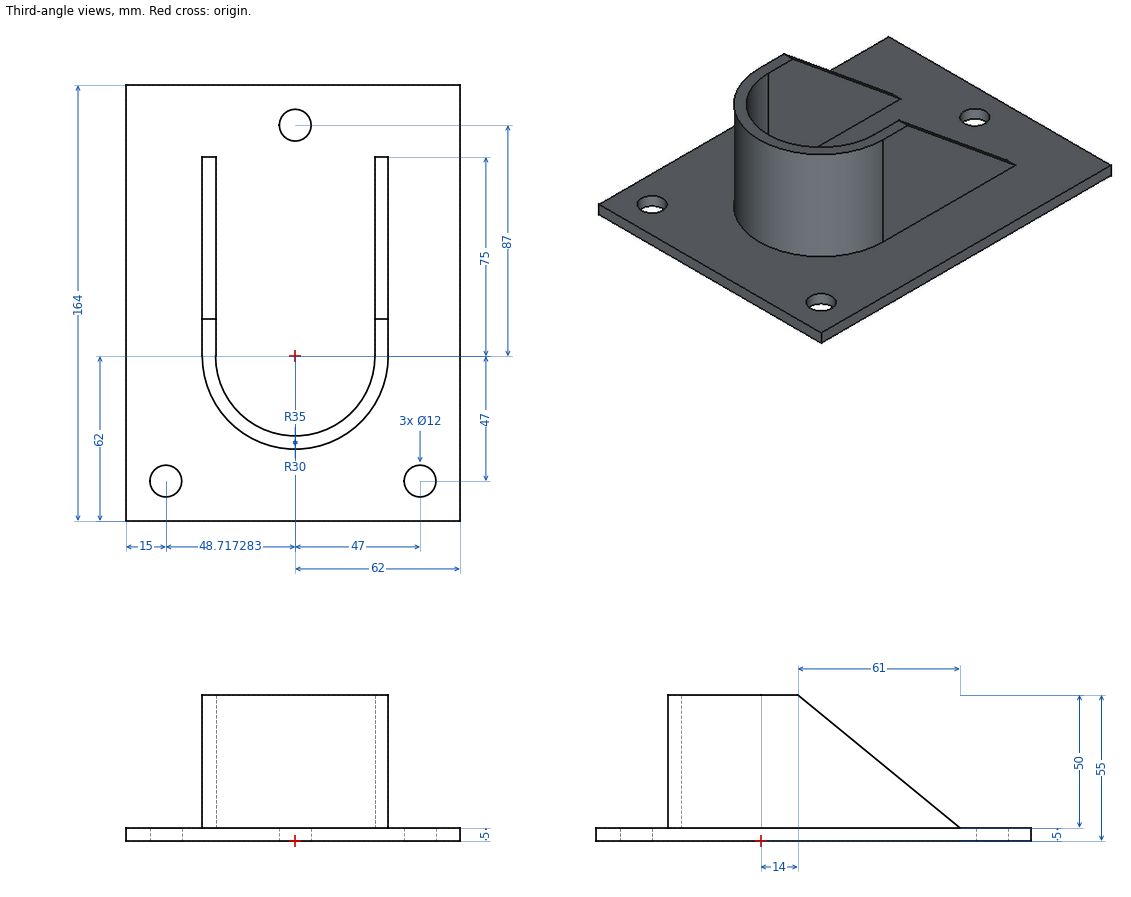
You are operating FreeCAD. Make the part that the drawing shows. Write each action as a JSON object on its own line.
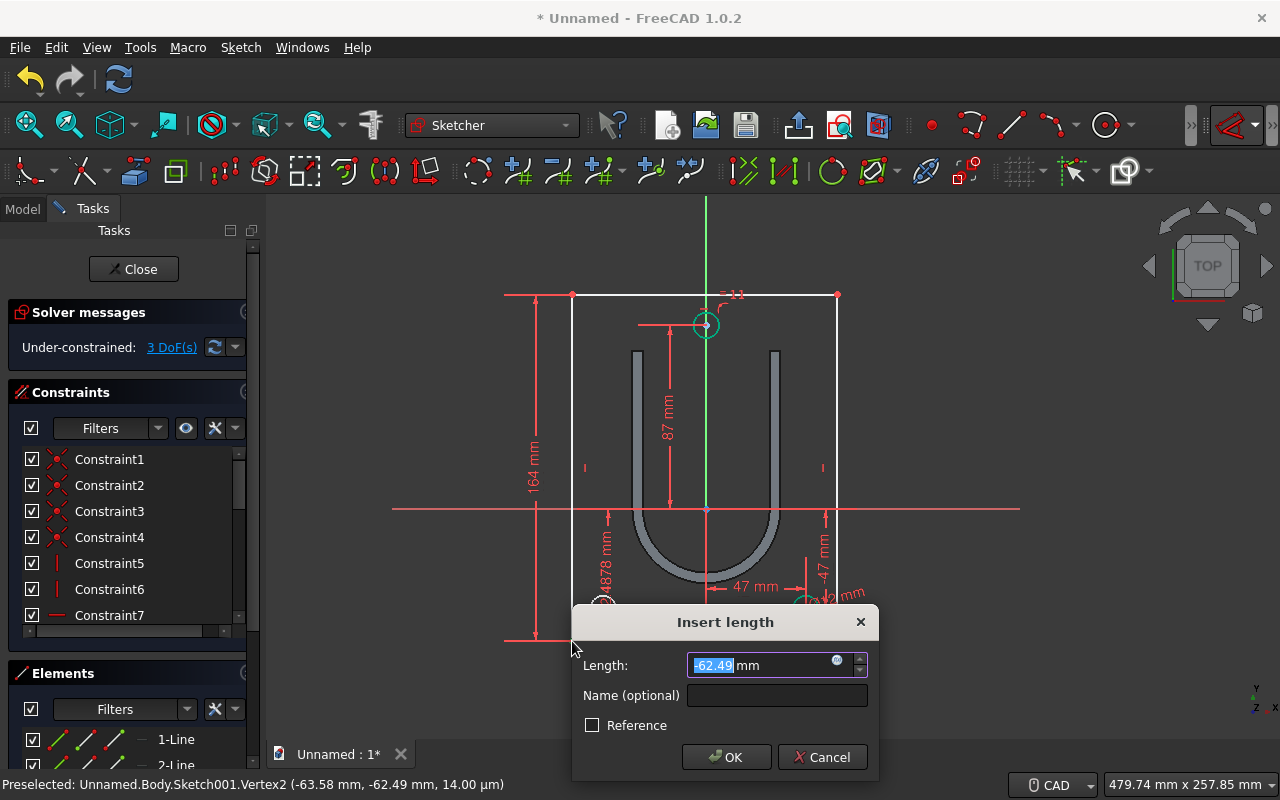
{"action": "type", "text": "-62"}
{"action": "key", "text": "Return"}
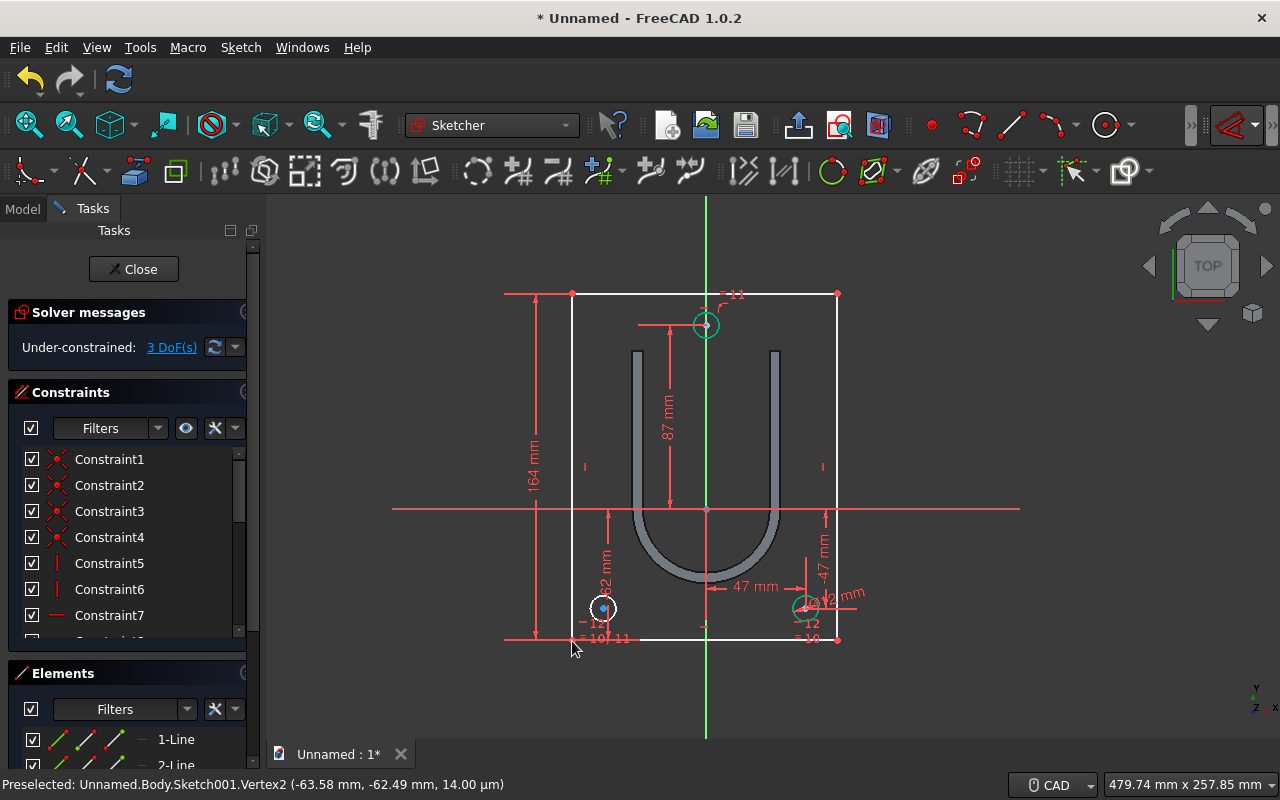
{"action": "left_click", "coordinate": [837, 640]}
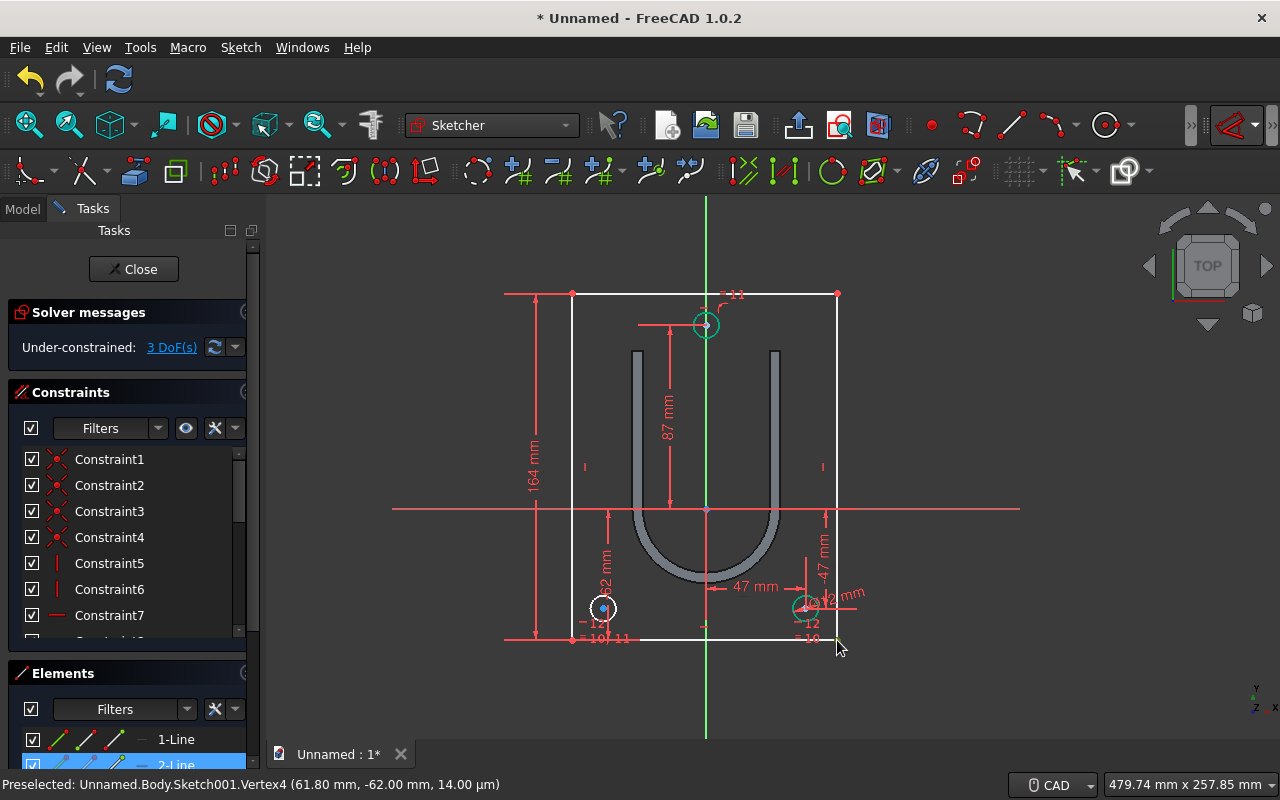
{"action": "left_click", "coordinate": [1258, 126]}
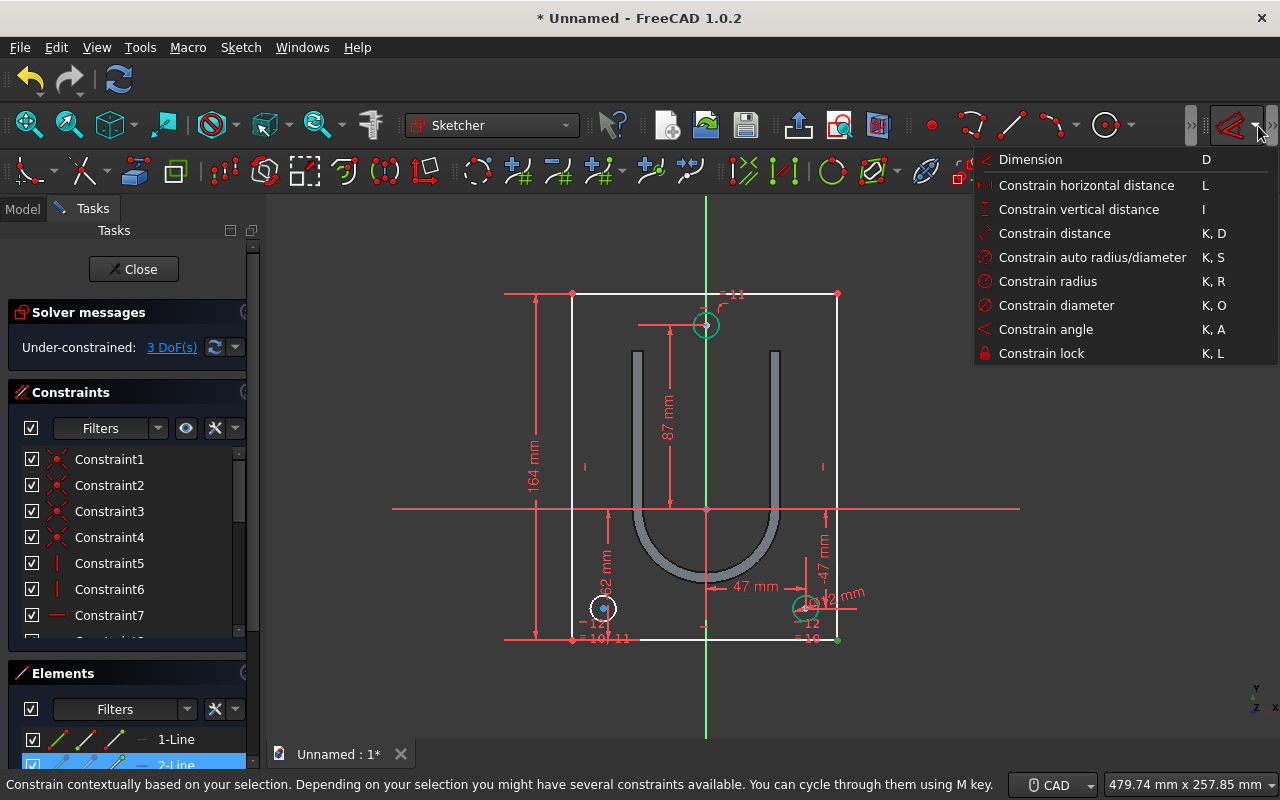
{"action": "left_click", "coordinate": [1126, 185]}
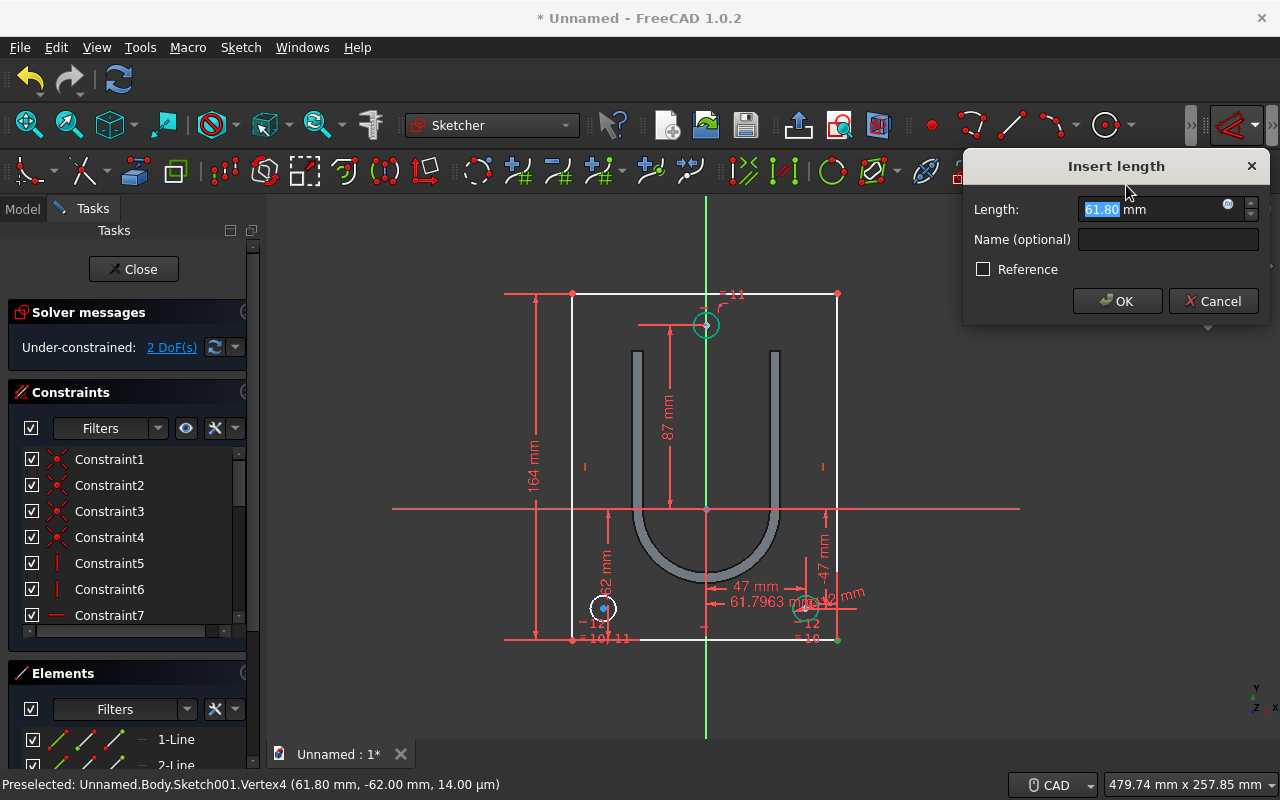
{"action": "type", "text": "62"}
{"action": "key", "text": "Return"}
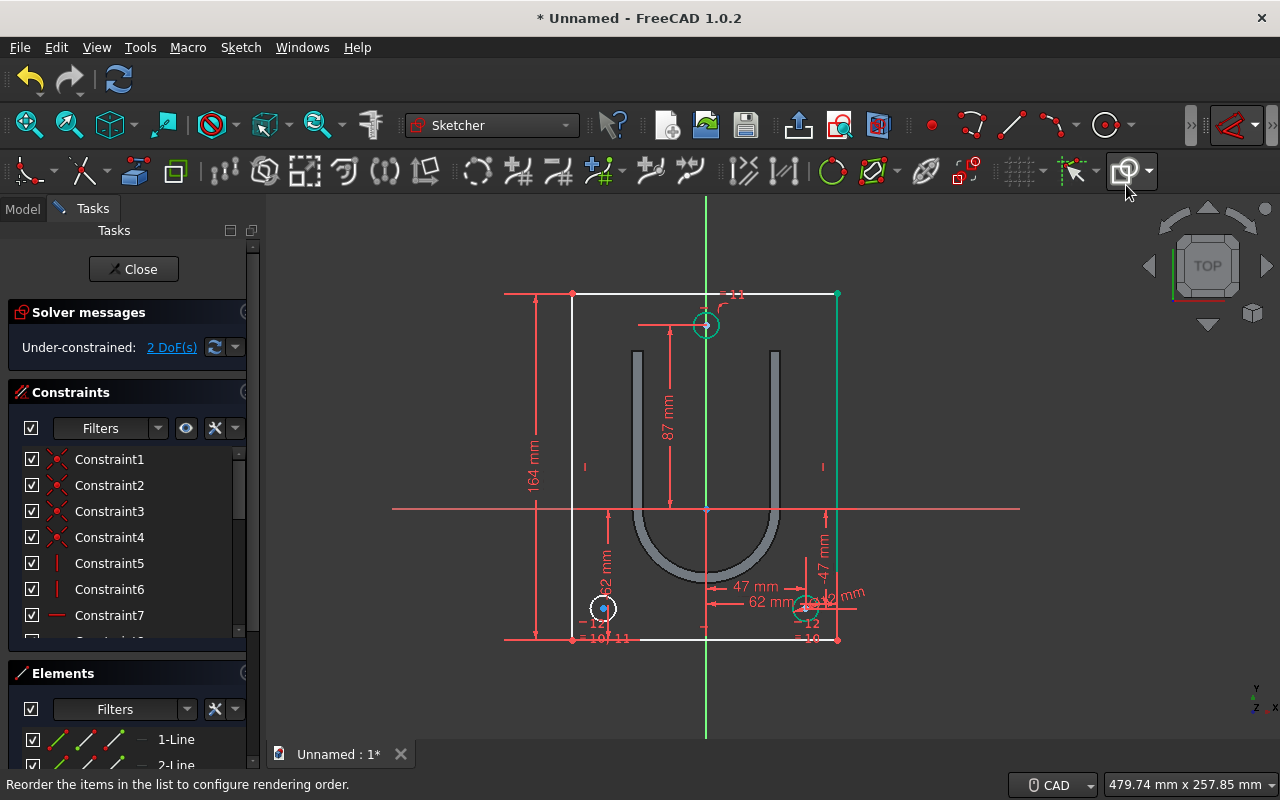
{"action": "scroll", "coordinate": [572, 640], "scroll_direction": "up", "scroll_amount": 2}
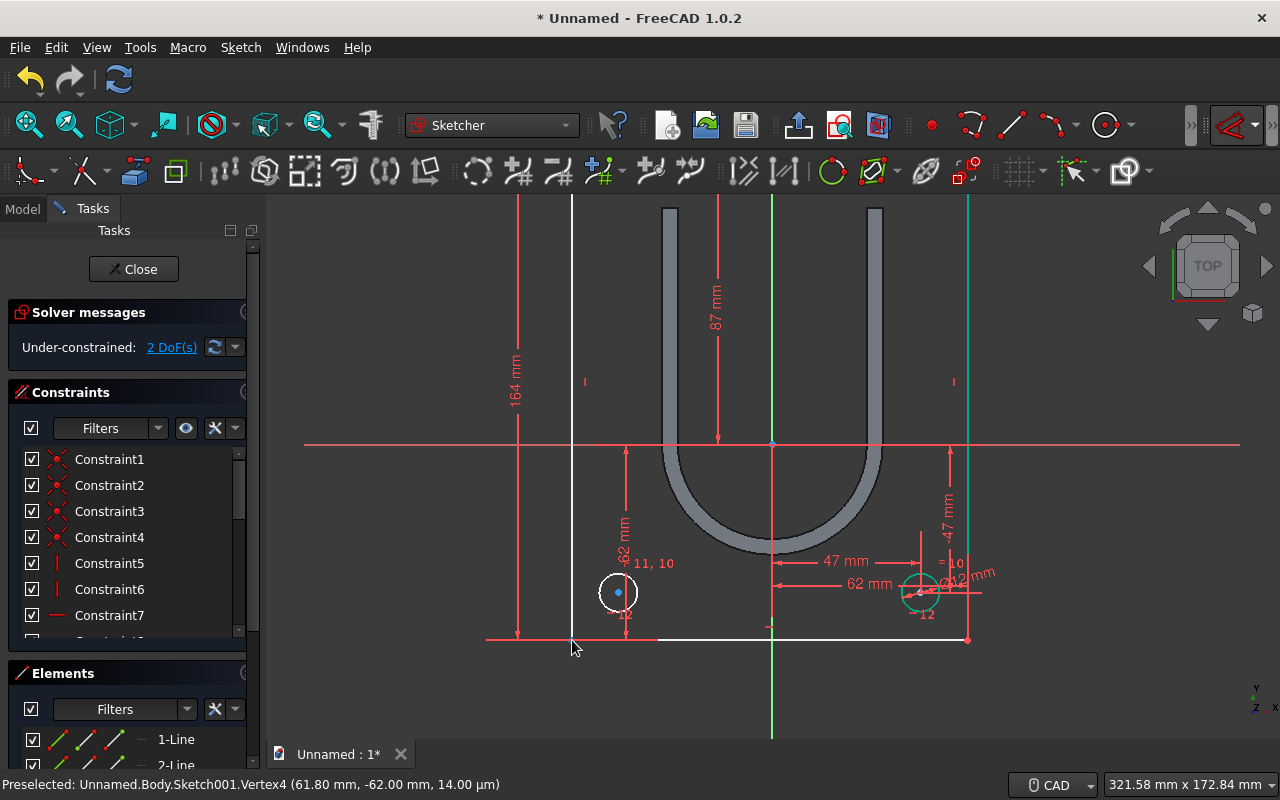
{"action": "left_click", "coordinate": [572, 640]}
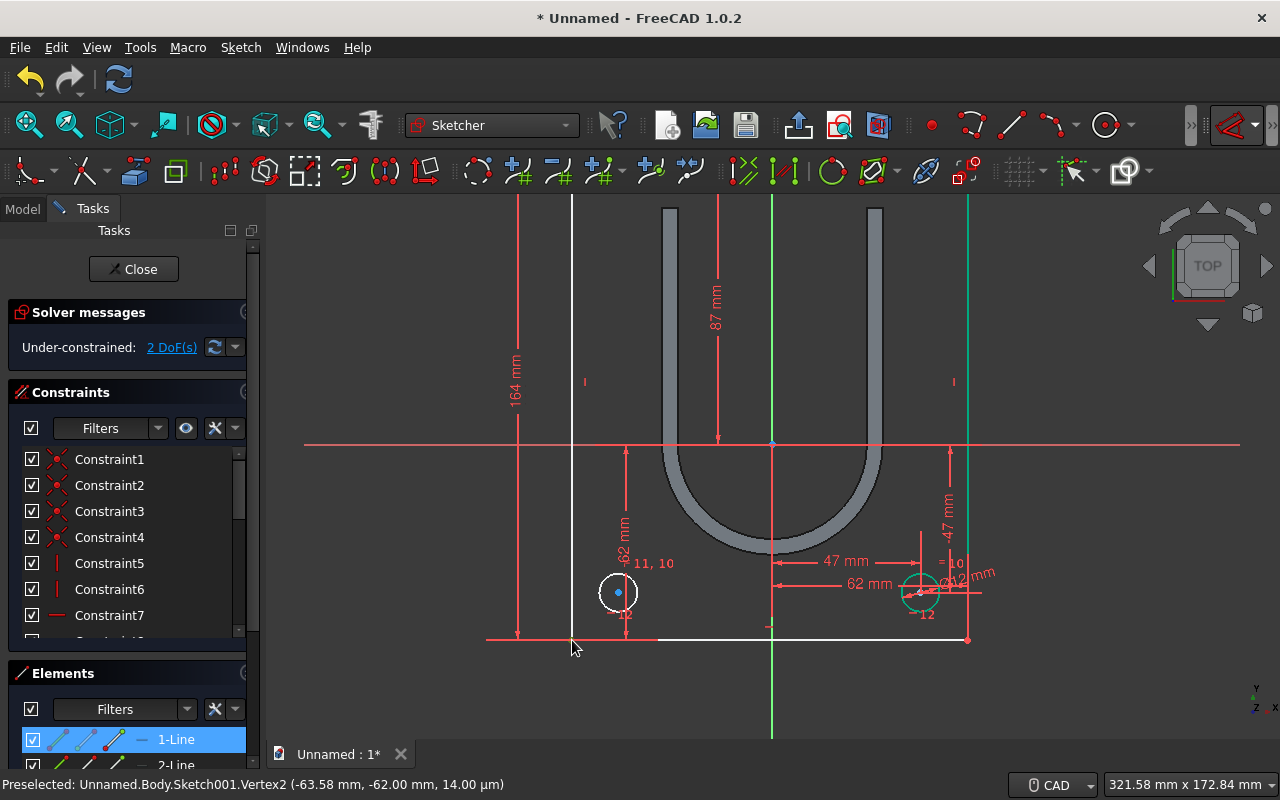
{"action": "left_click", "coordinate": [618, 593]}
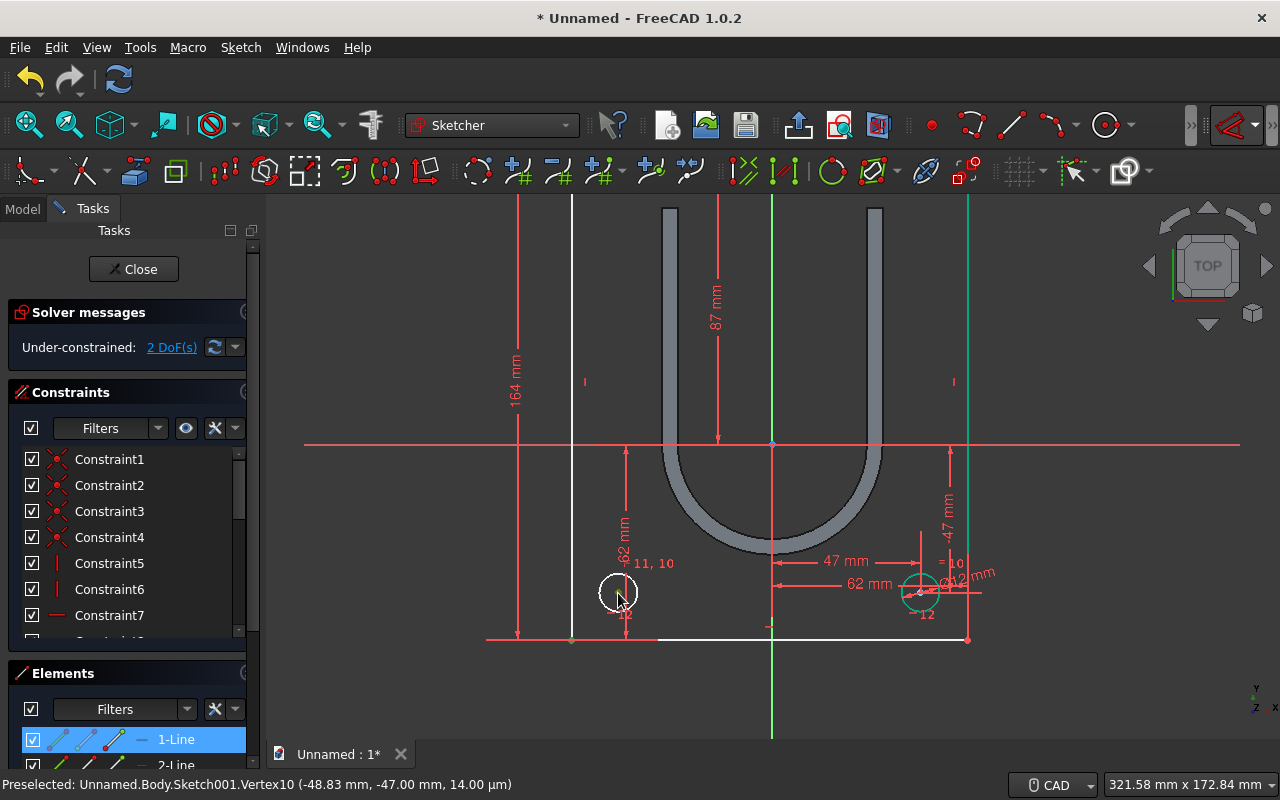
{"action": "key", "text": "l"}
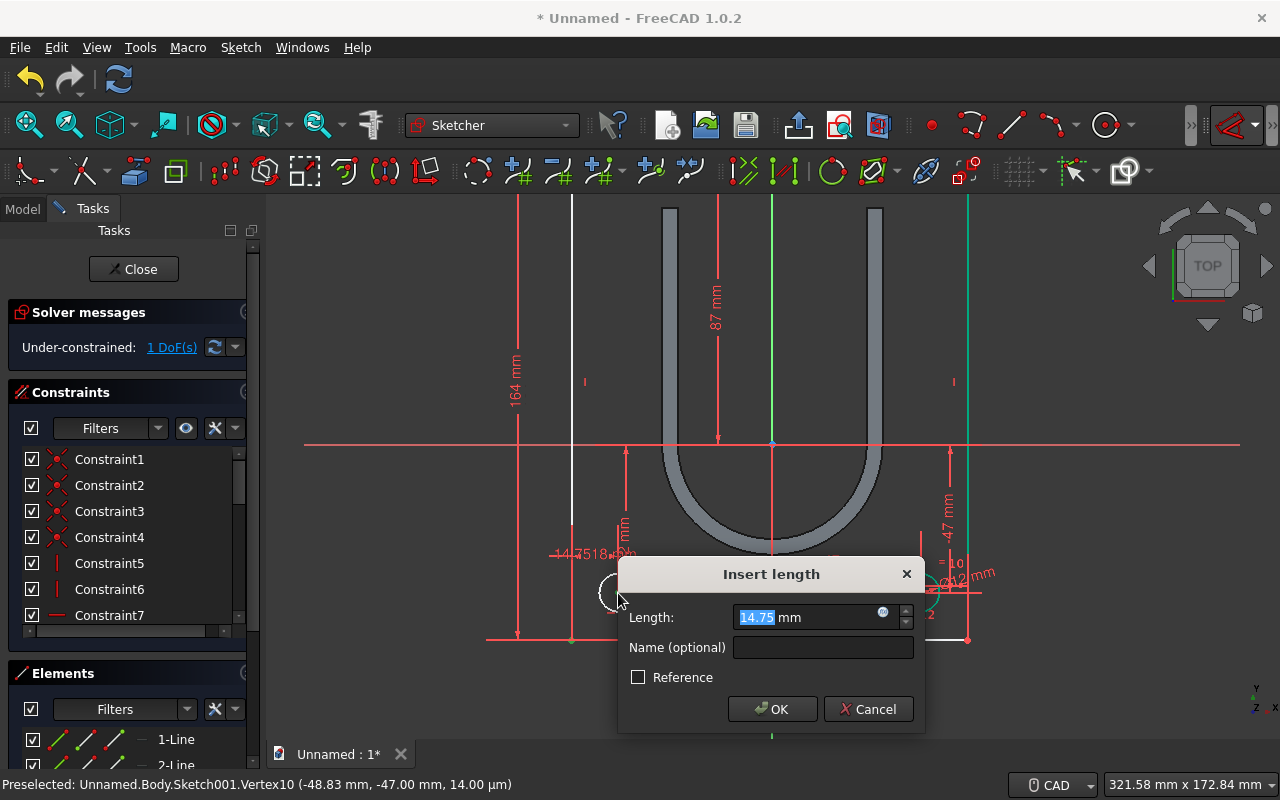
{"action": "type", "text": "15"}
{"action": "key", "text": "Return"}